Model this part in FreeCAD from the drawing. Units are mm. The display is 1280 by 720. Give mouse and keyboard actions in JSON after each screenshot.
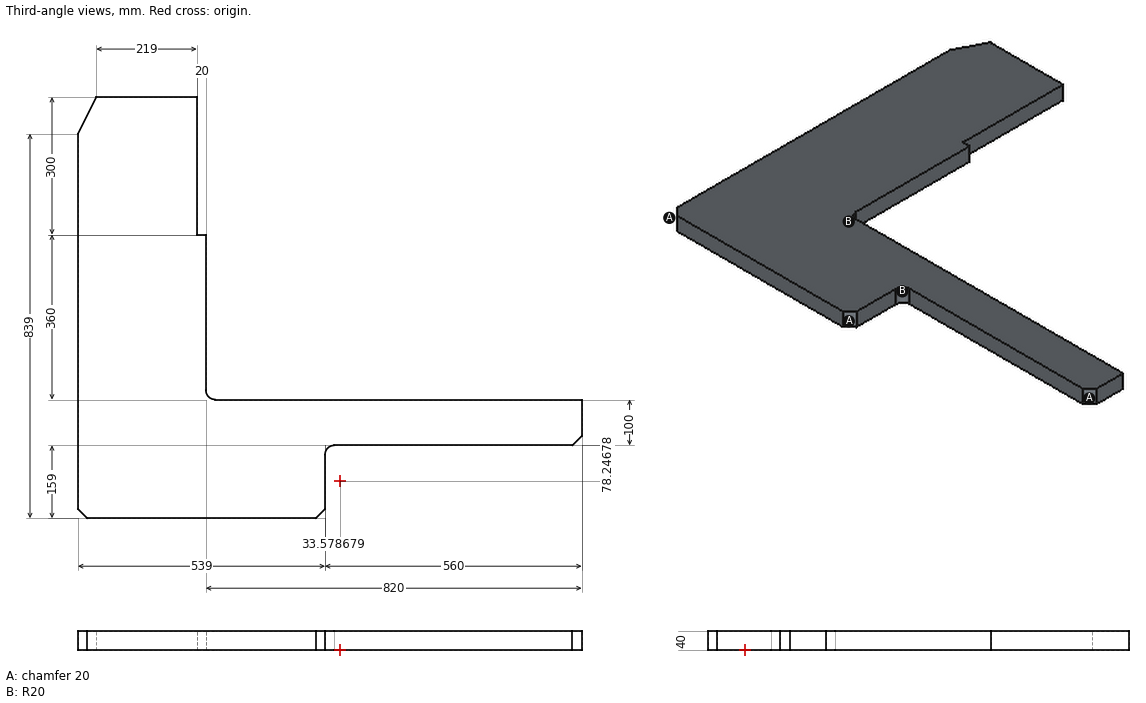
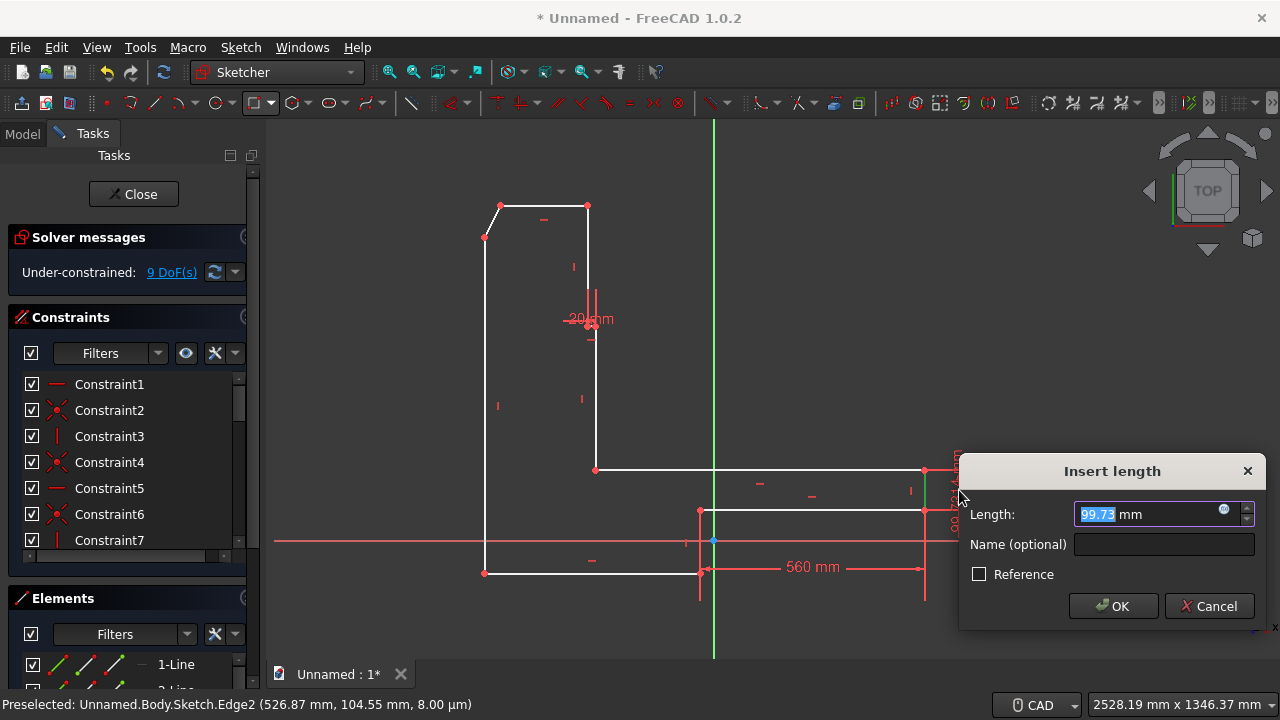
{"action": "type", "text": "100"}
{"action": "key", "text": "Return"}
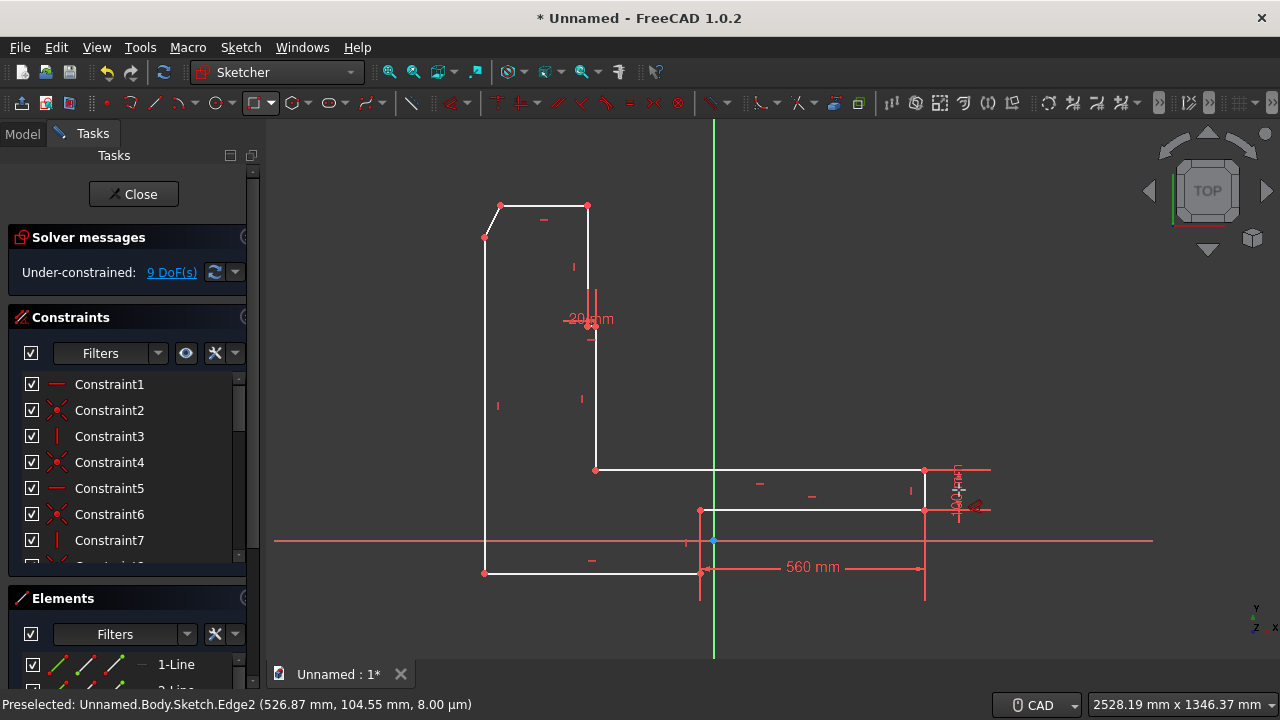
{"action": "left_click", "coordinate": [826, 470]}
{"action": "left_click", "coordinate": [685, 504]}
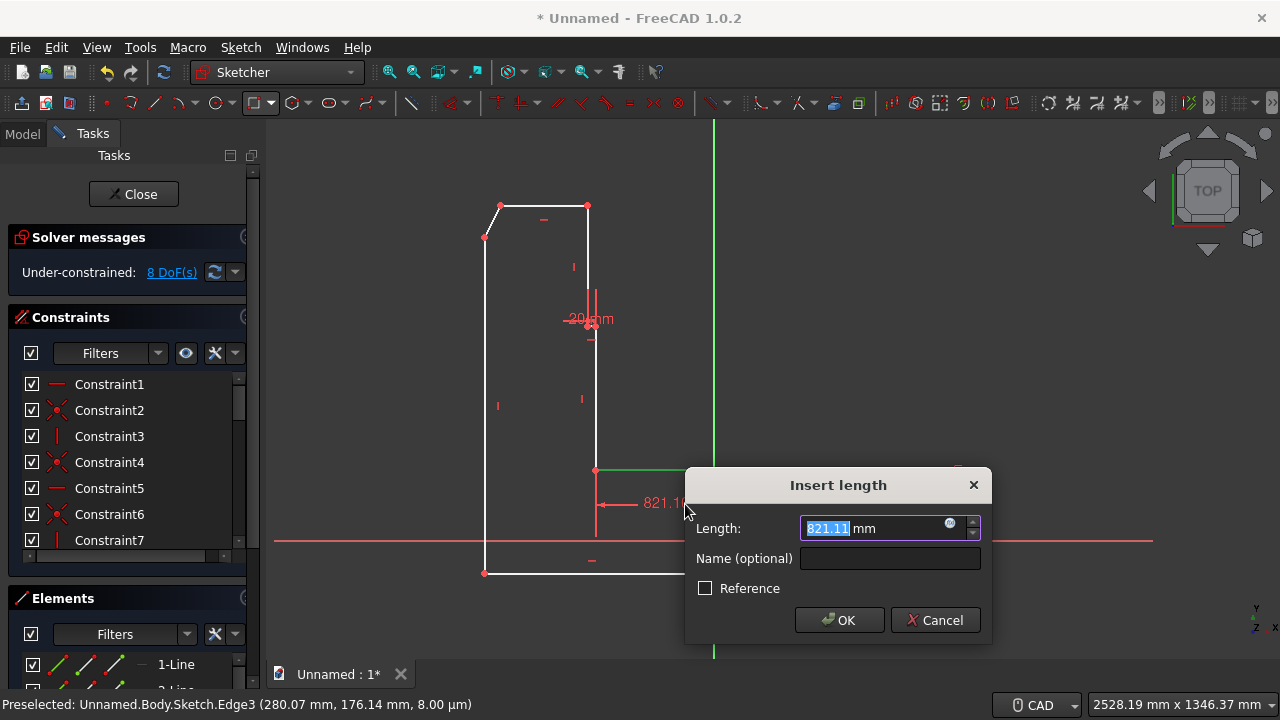
{"action": "type", "text": "820"}
{"action": "key", "text": "Return"}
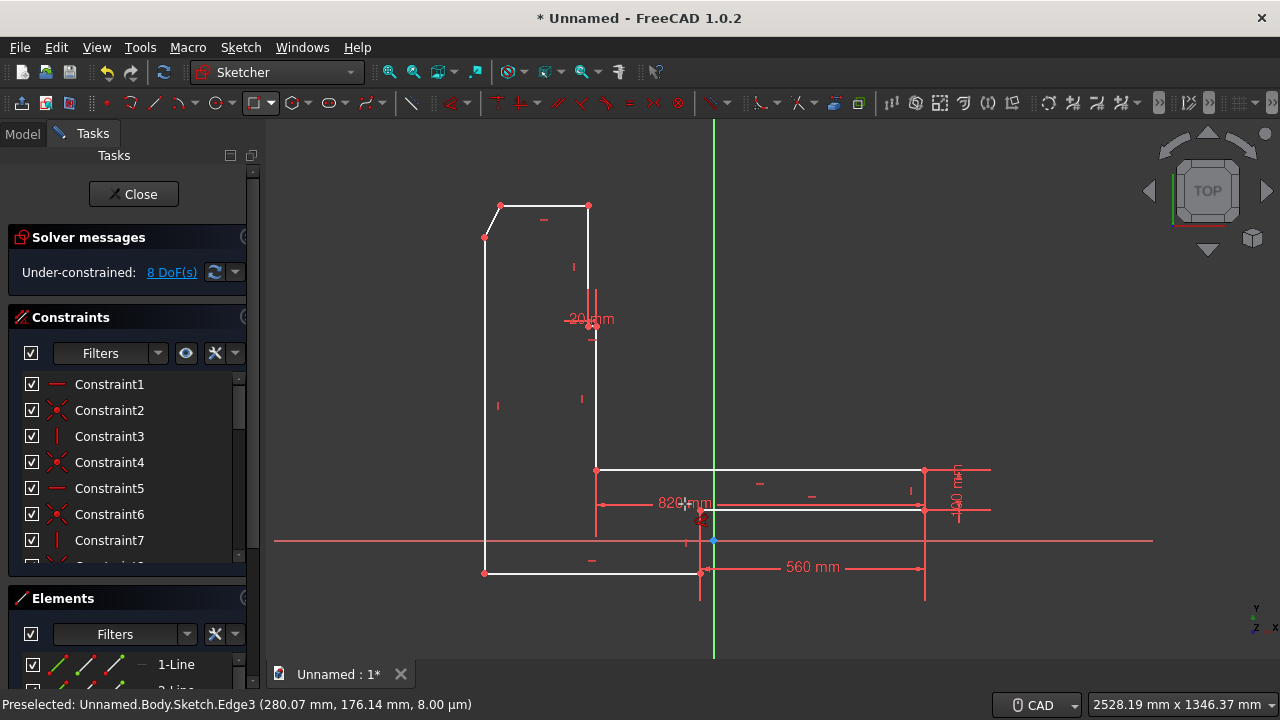
{"action": "left_click", "coordinate": [596, 427]}
{"action": "left_click", "coordinate": [562, 398]}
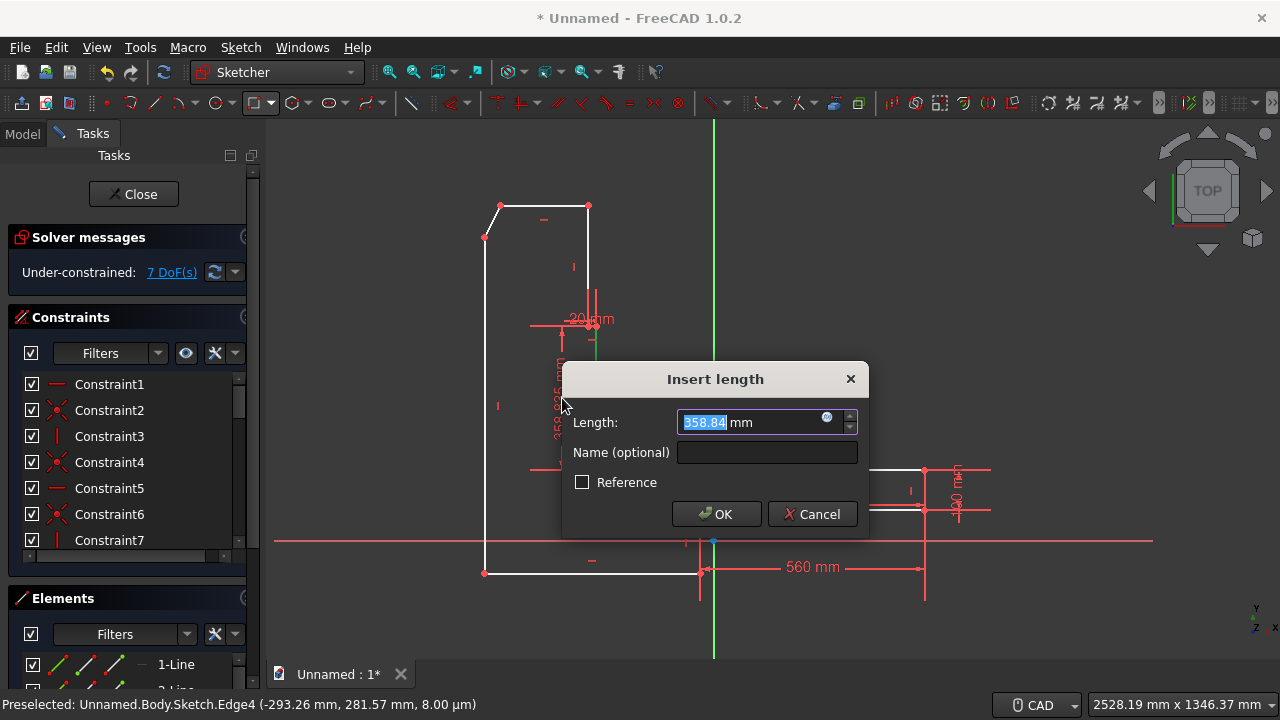
{"action": "type", "text": "360"}
{"action": "key", "text": "Return"}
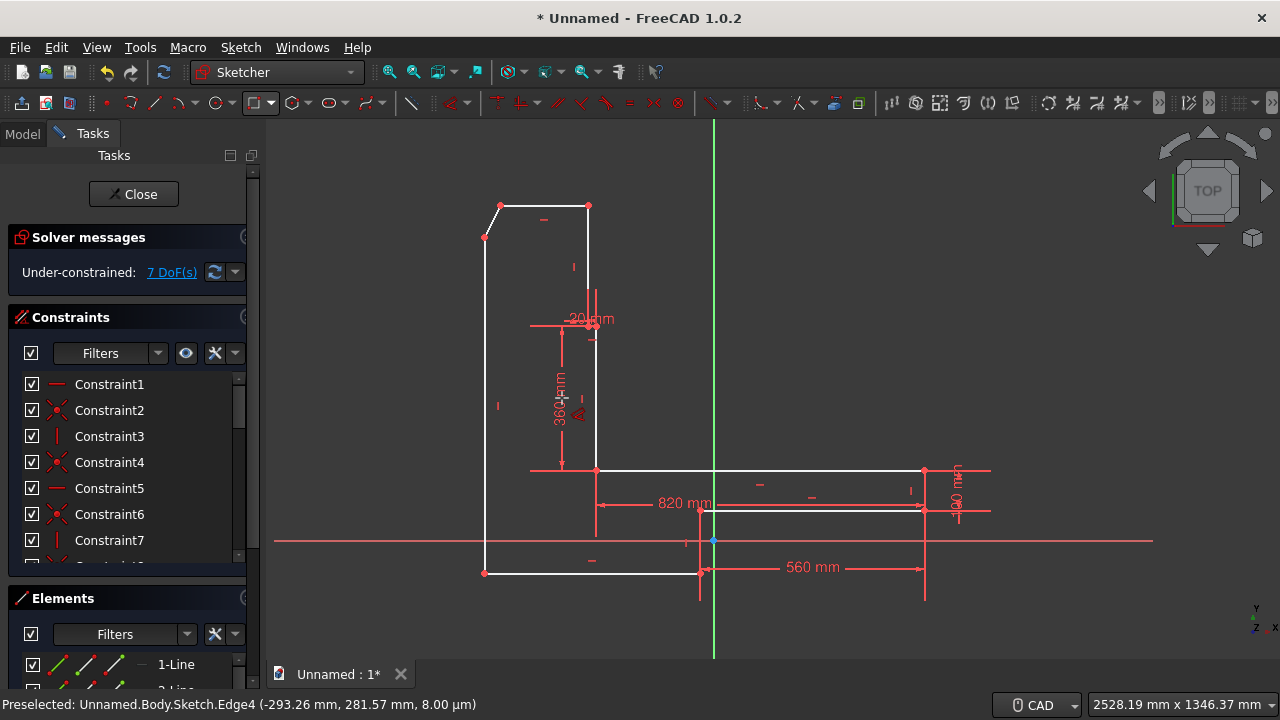
{"action": "left_click", "coordinate": [588, 290]}
{"action": "left_click", "coordinate": [554, 266]}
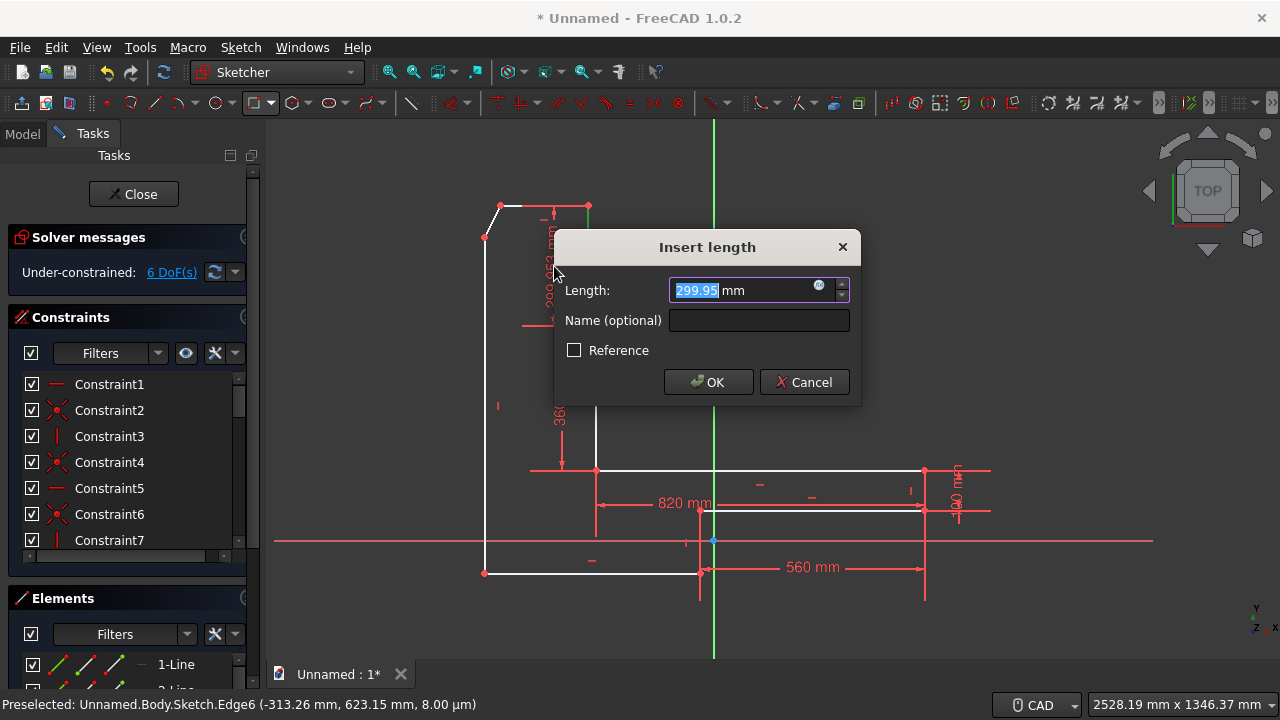
{"action": "type", "text": "300"}
{"action": "key", "text": "Return"}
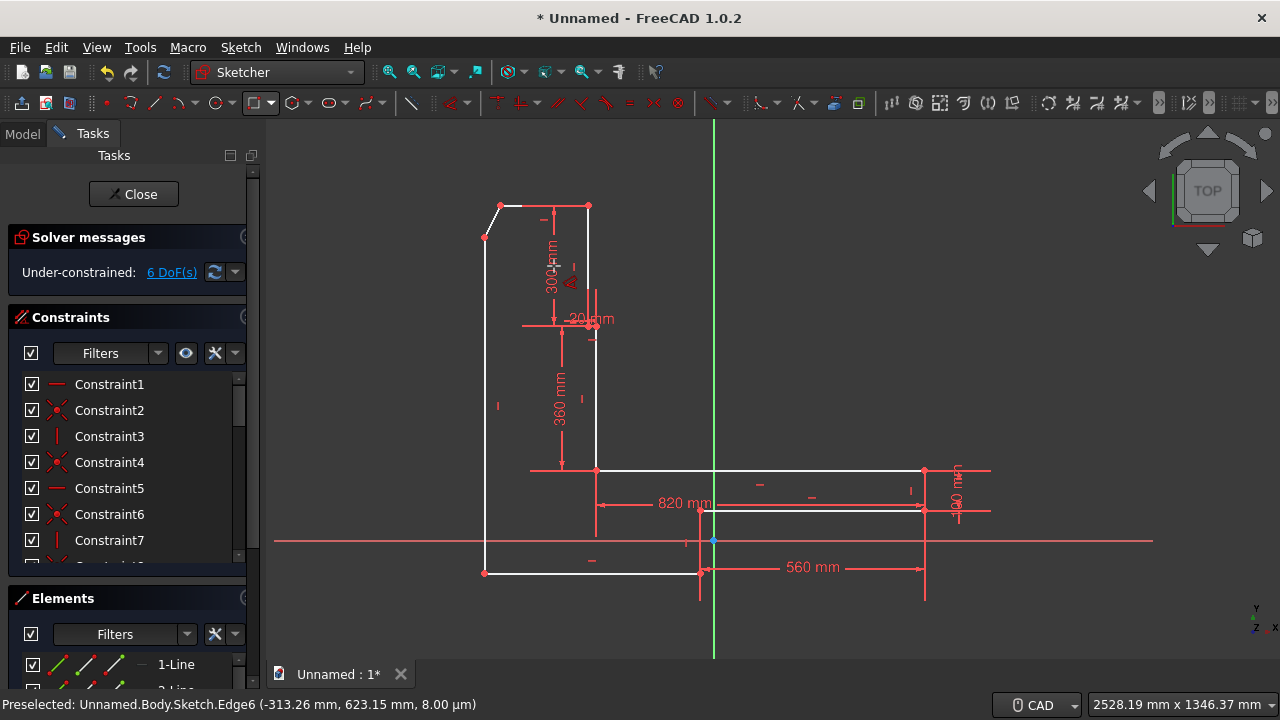
{"action": "left_click", "coordinate": [562, 206]}
{"action": "left_click", "coordinate": [544, 172]}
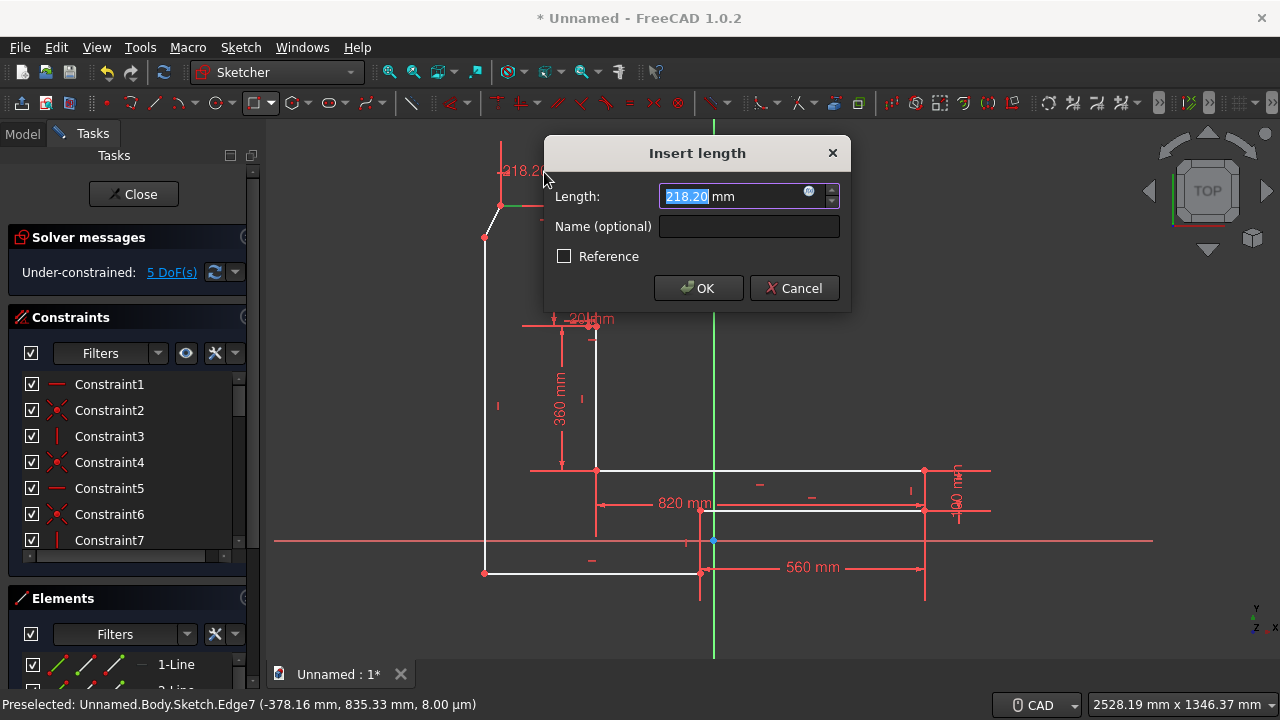
{"action": "type", "text": "219"}
{"action": "key", "text": "Return"}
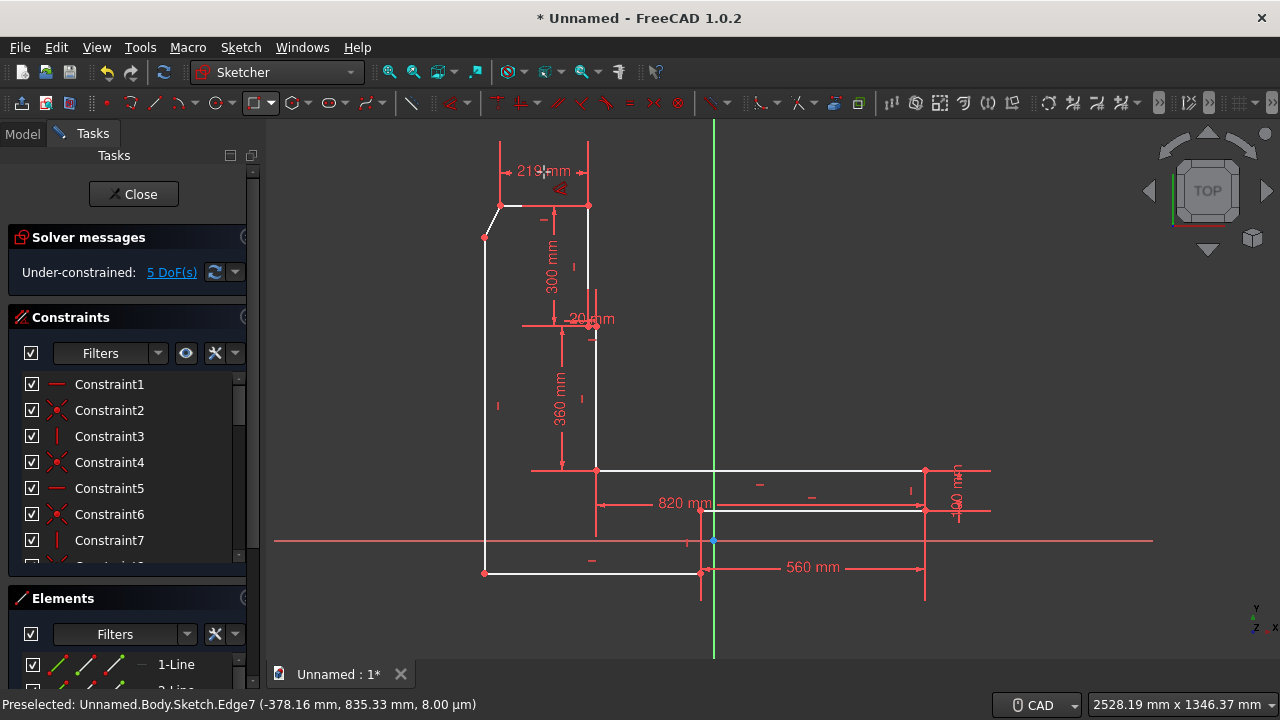
{"action": "left_click", "coordinate": [485, 339]}
{"action": "left_click", "coordinate": [451, 406]}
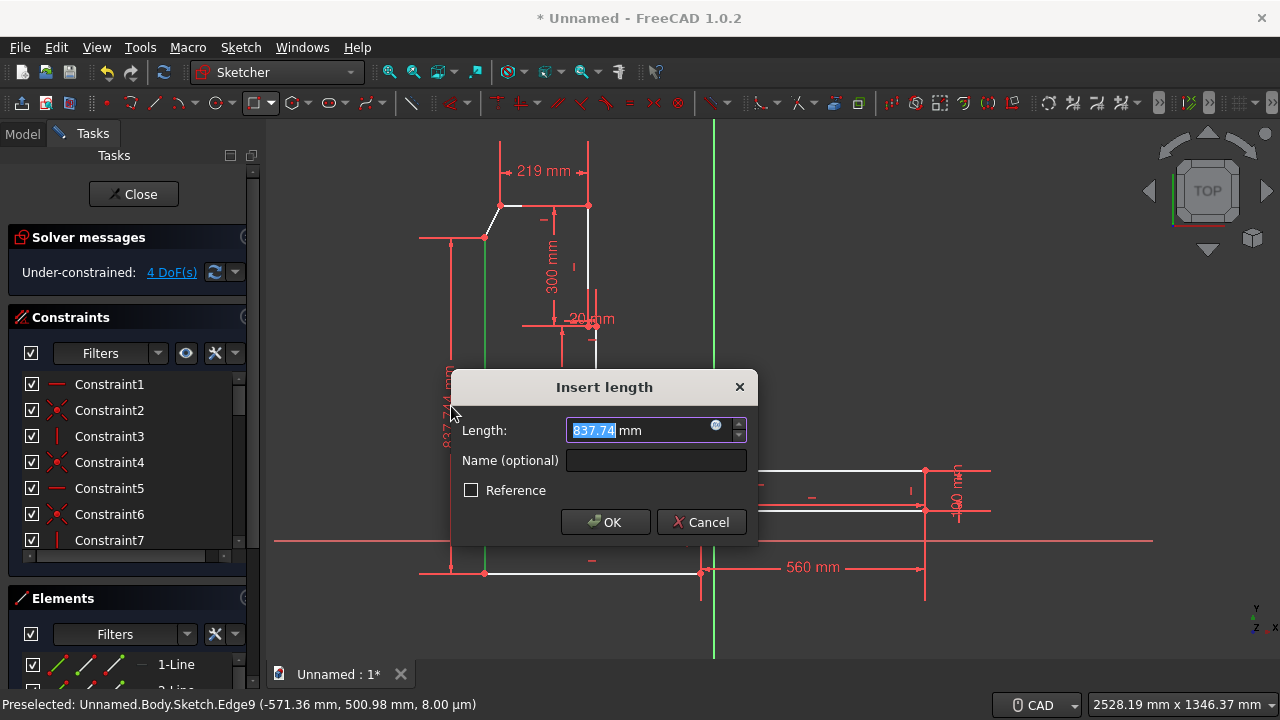
{"action": "type", "text": "839"}
{"action": "key", "text": "Return"}